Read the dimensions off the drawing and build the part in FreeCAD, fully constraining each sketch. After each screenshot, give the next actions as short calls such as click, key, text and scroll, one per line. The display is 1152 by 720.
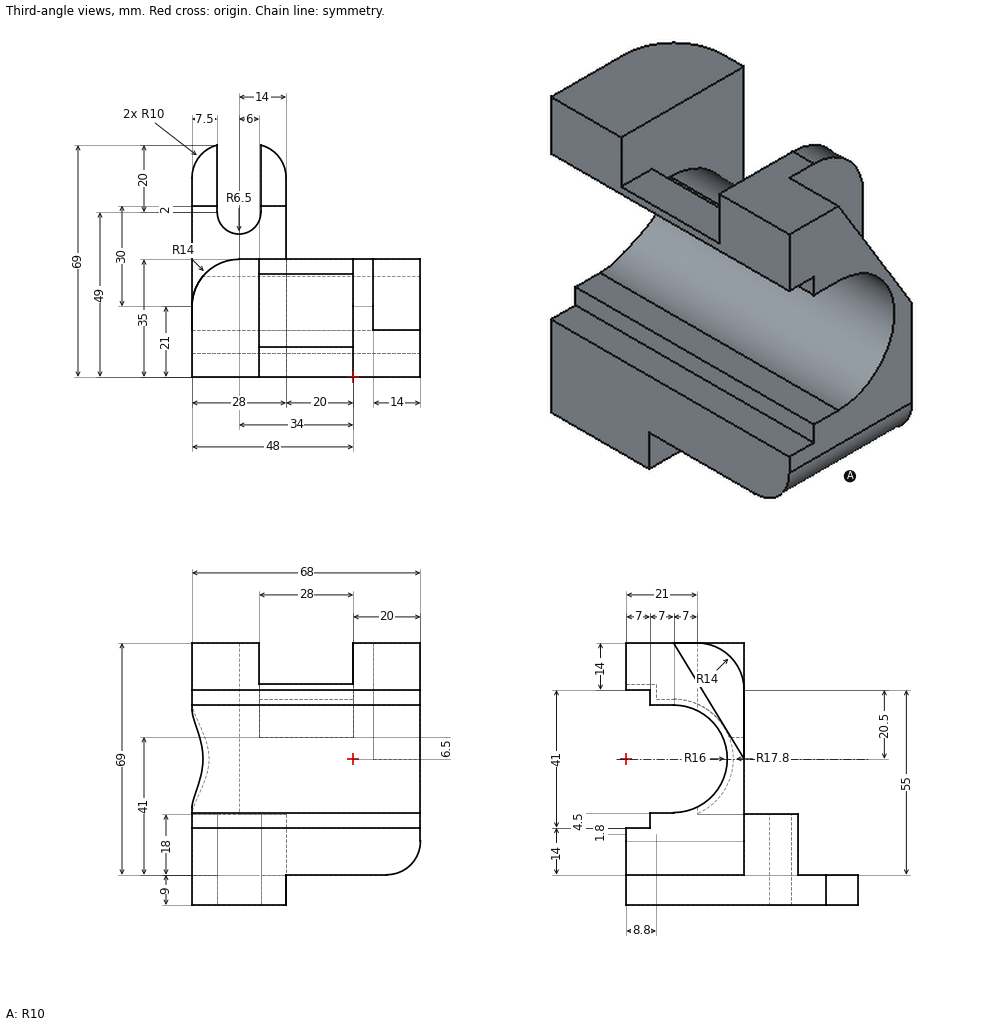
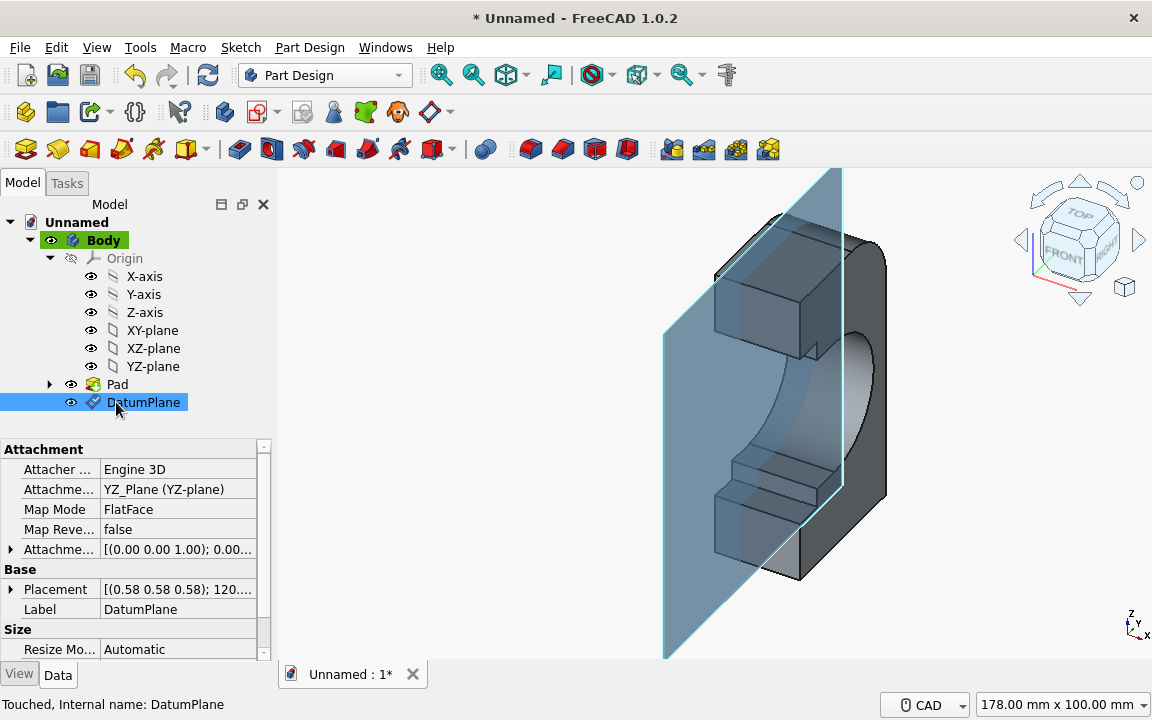
click(258, 112)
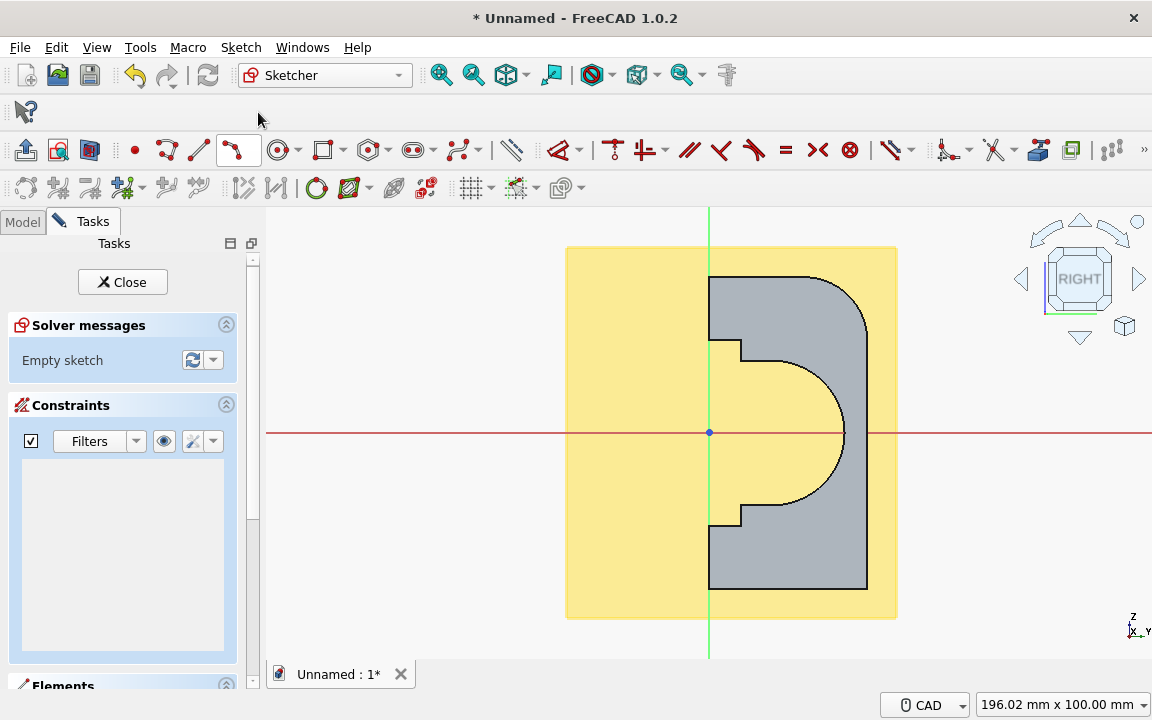
click(90, 150)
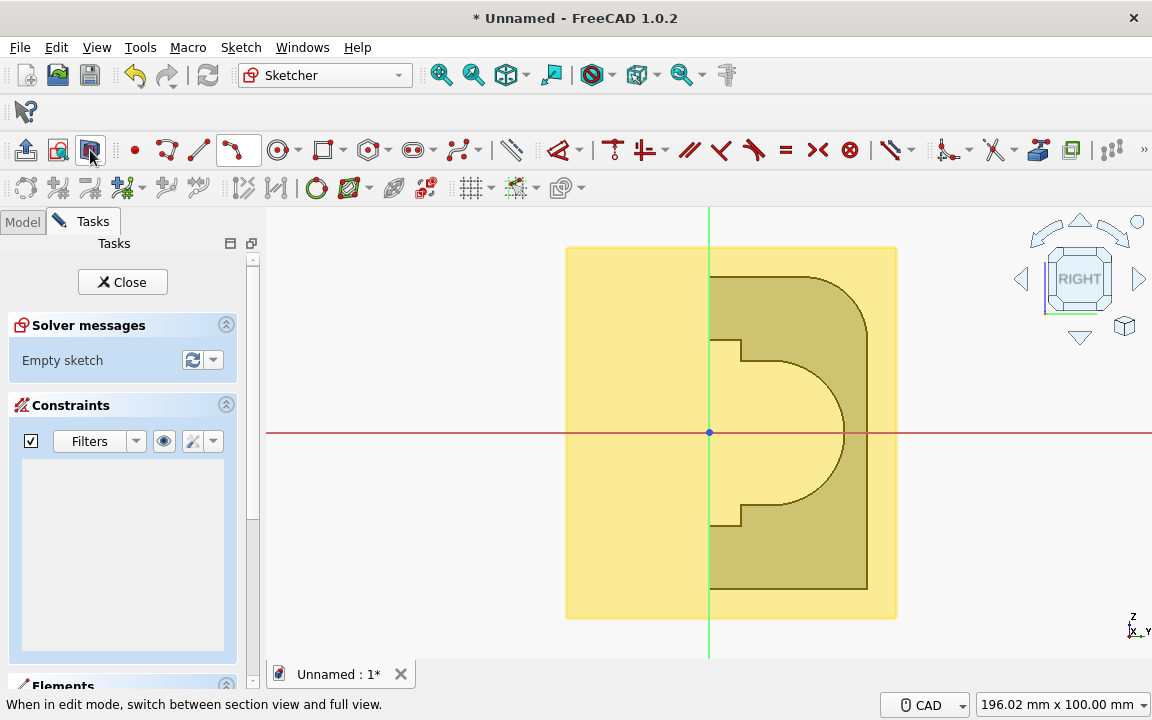
scroll(968, 260, up, 3)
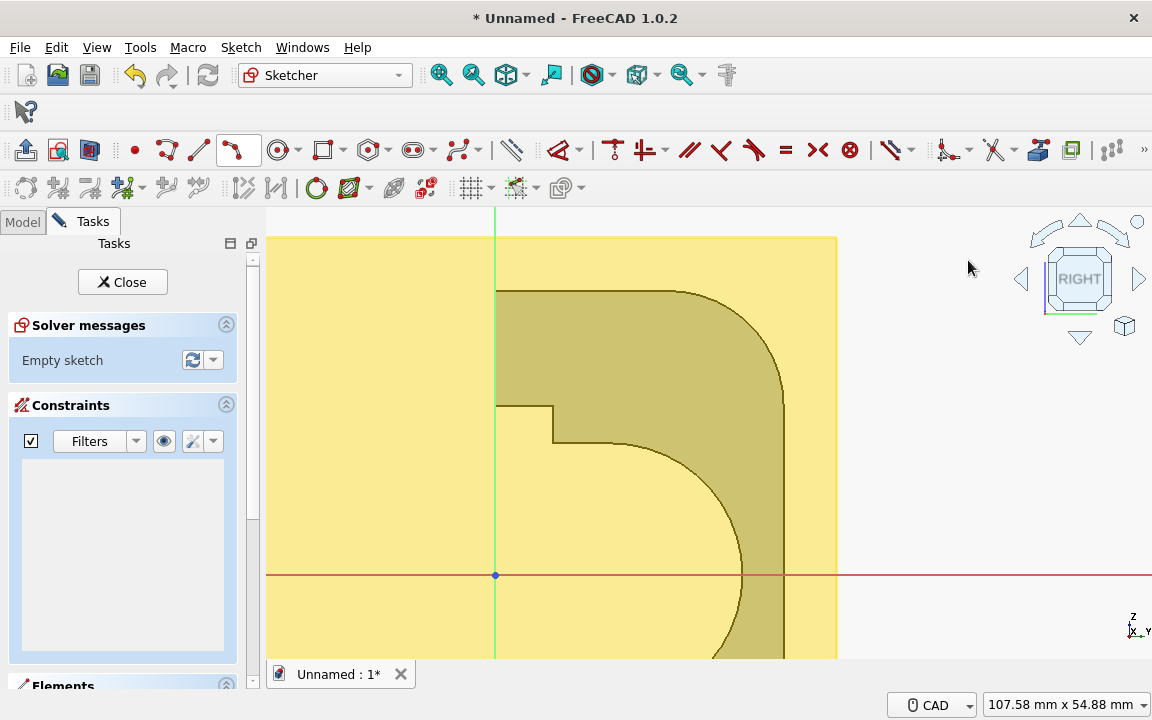
click(168, 150)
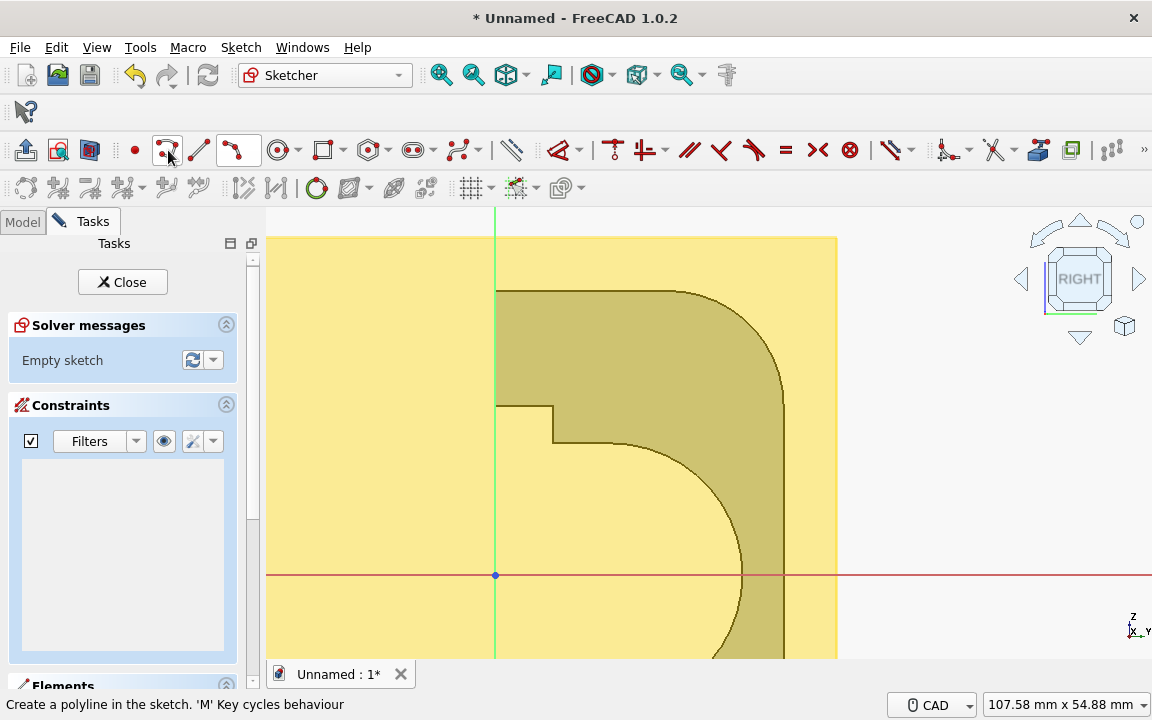
click(668, 291)
click(611, 291)
click(784, 575)
click(784, 406)
right_click(784, 406)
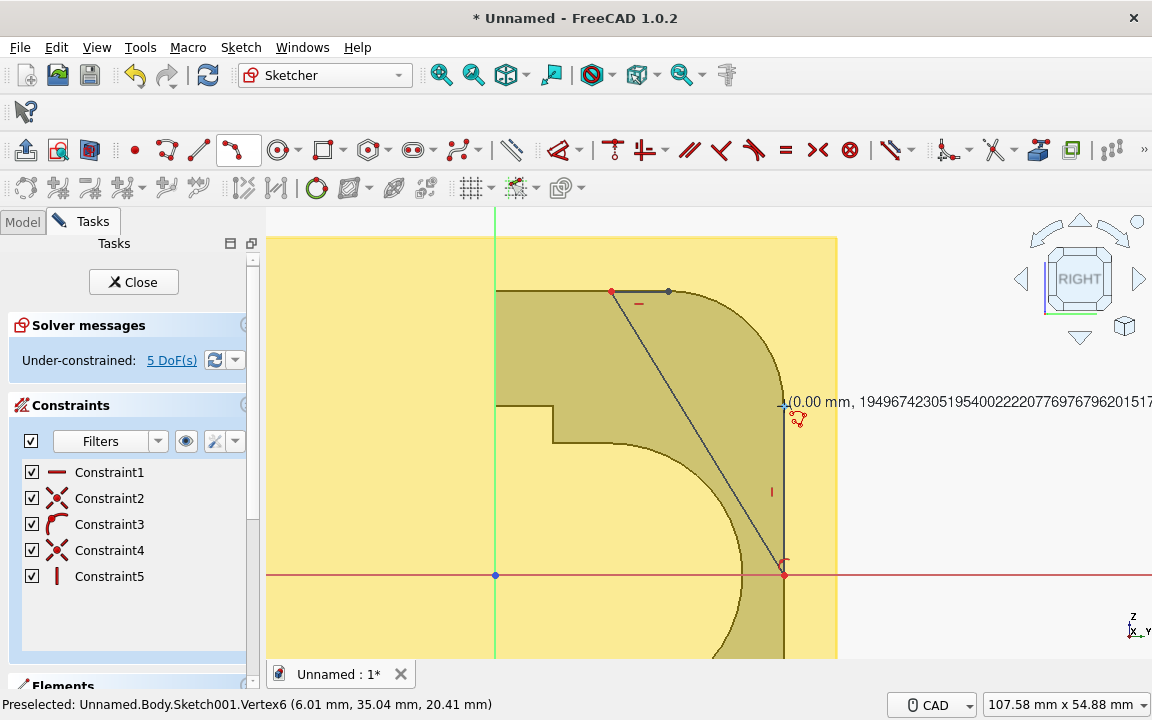
click(232, 150)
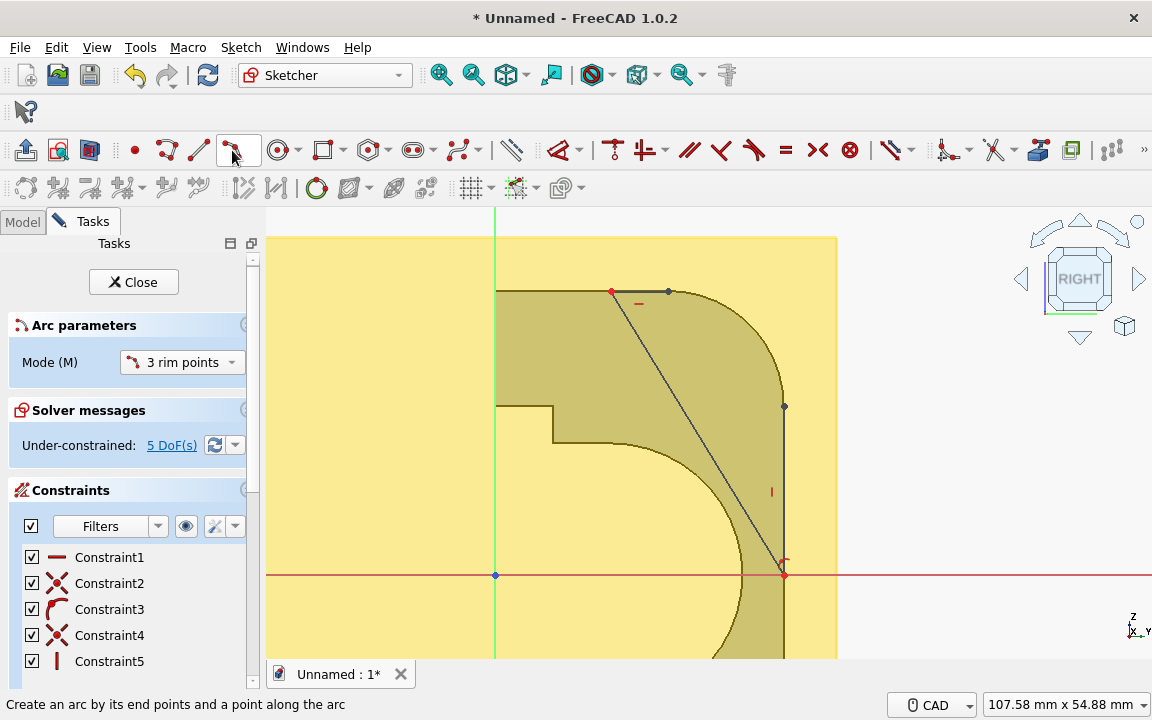
click(784, 407)
click(668, 292)
click(750, 325)
key(Escape)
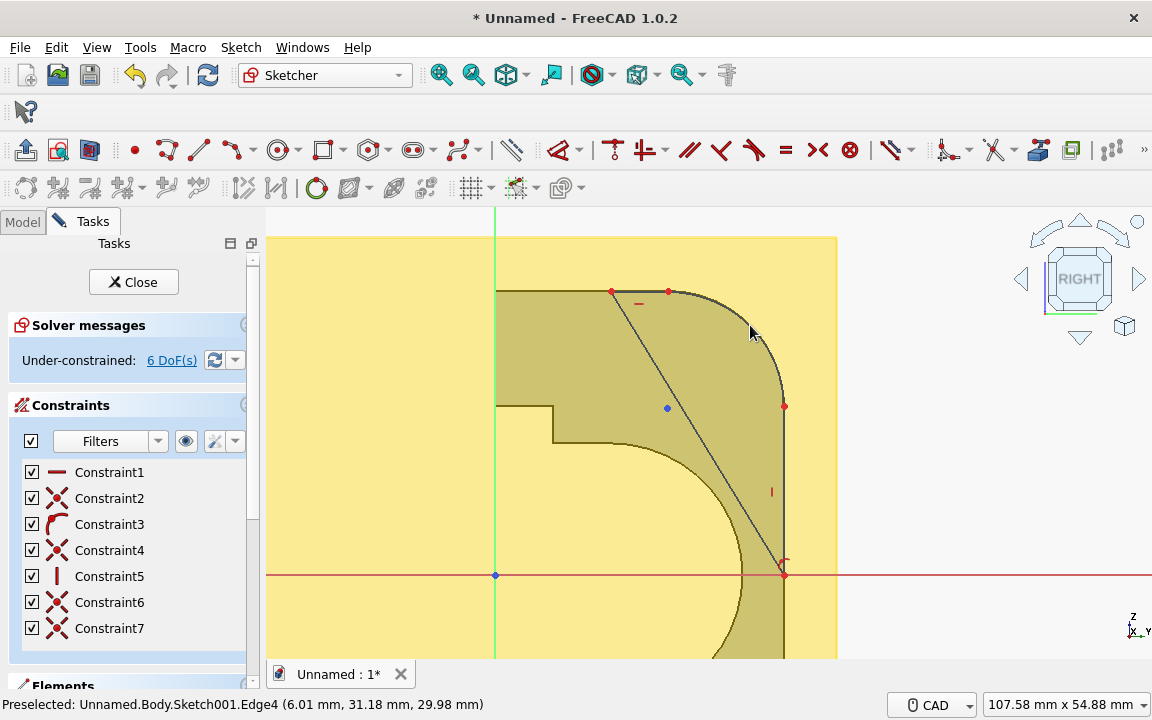
click(651, 292)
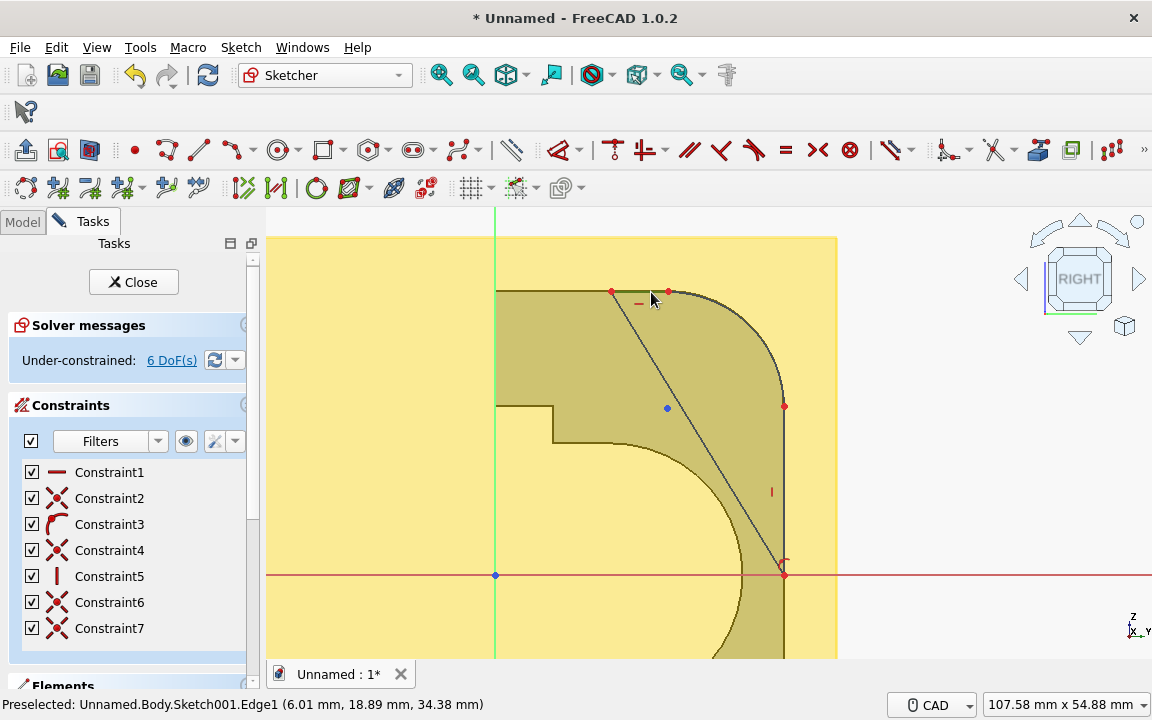
click(771, 355)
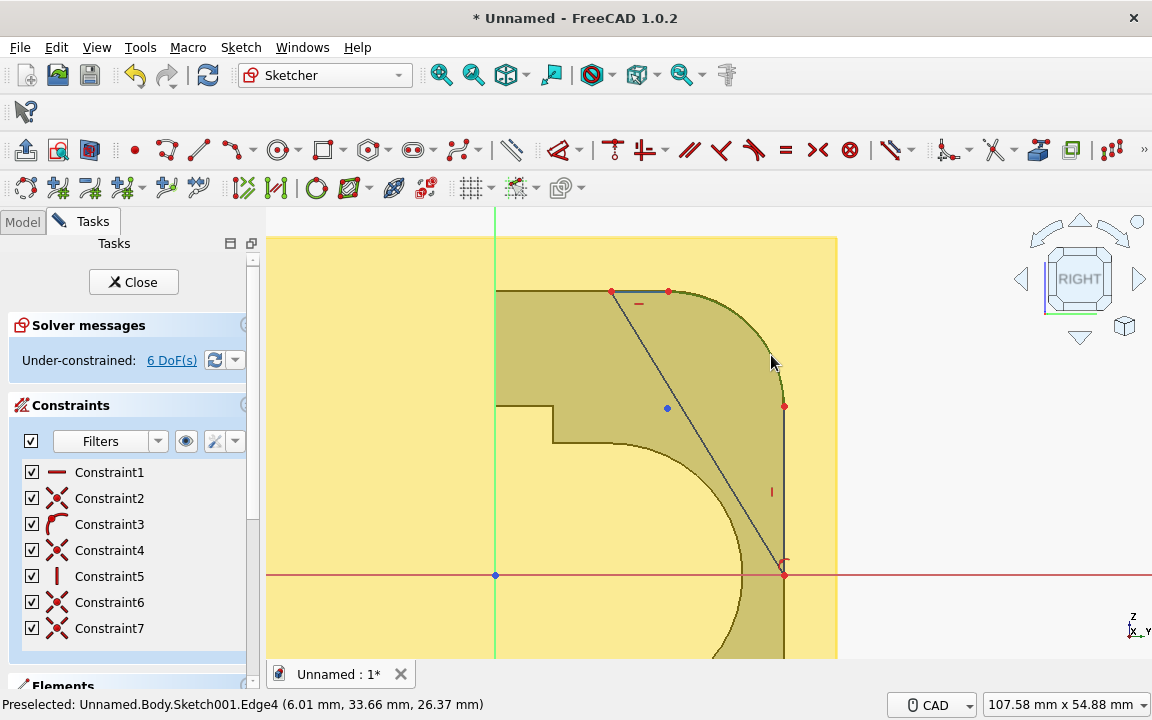
key(t)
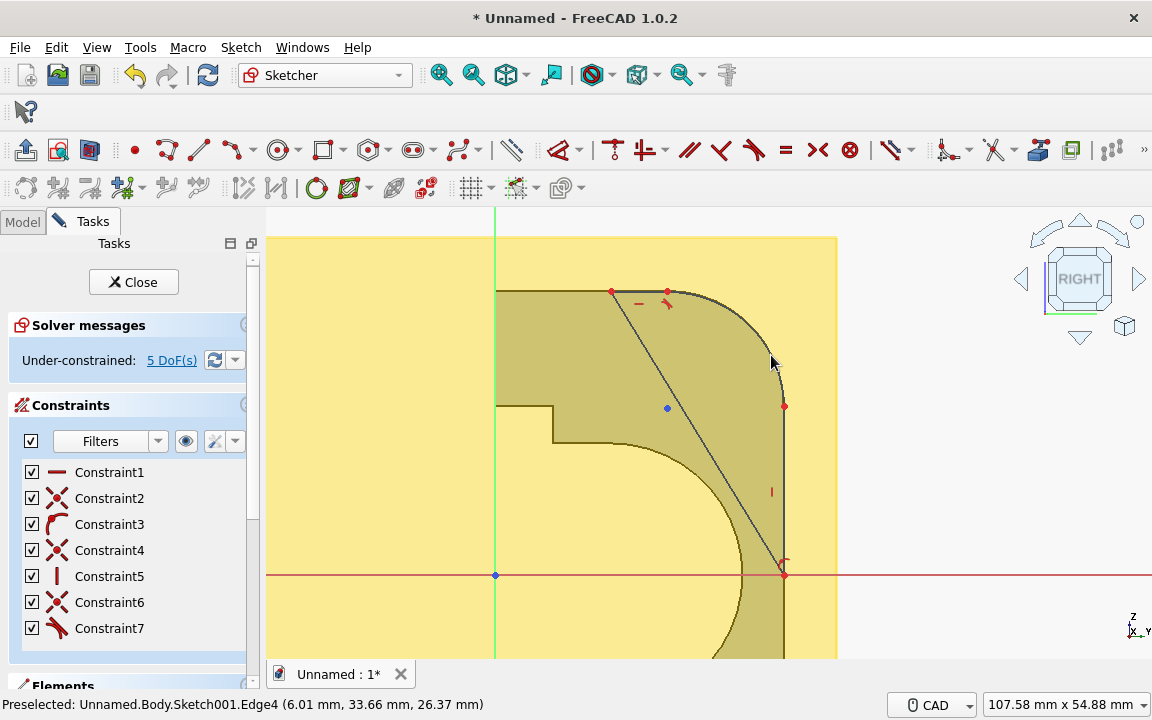
click(784, 525)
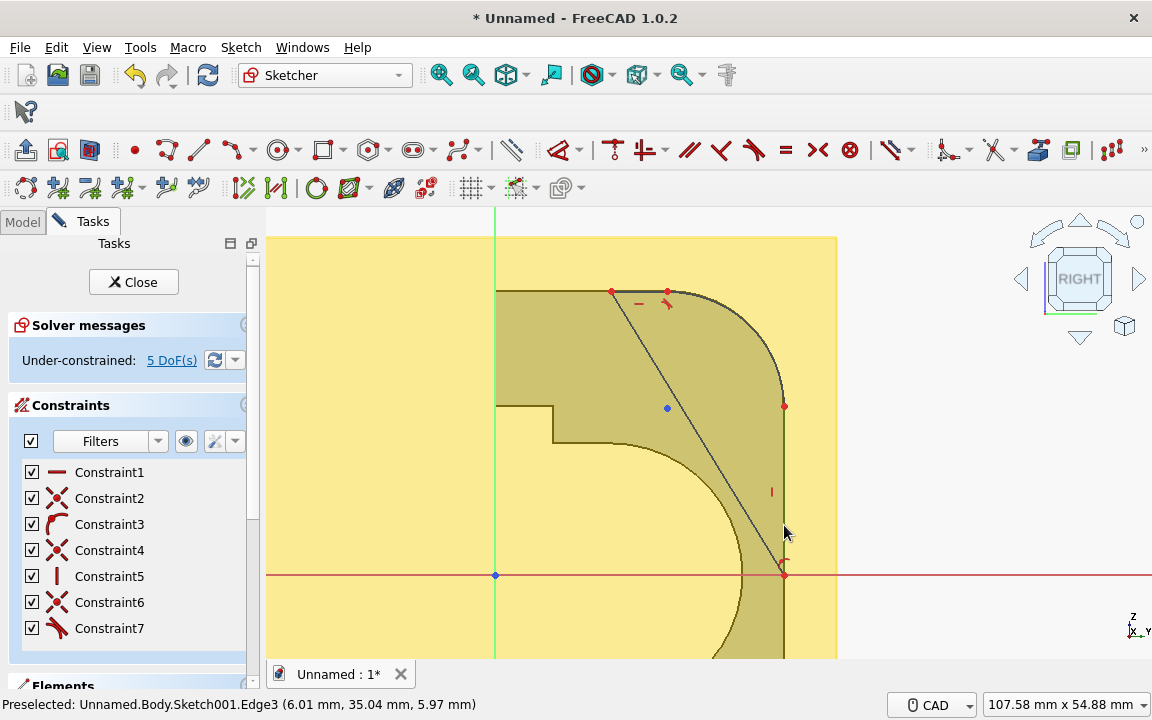
click(771, 355)